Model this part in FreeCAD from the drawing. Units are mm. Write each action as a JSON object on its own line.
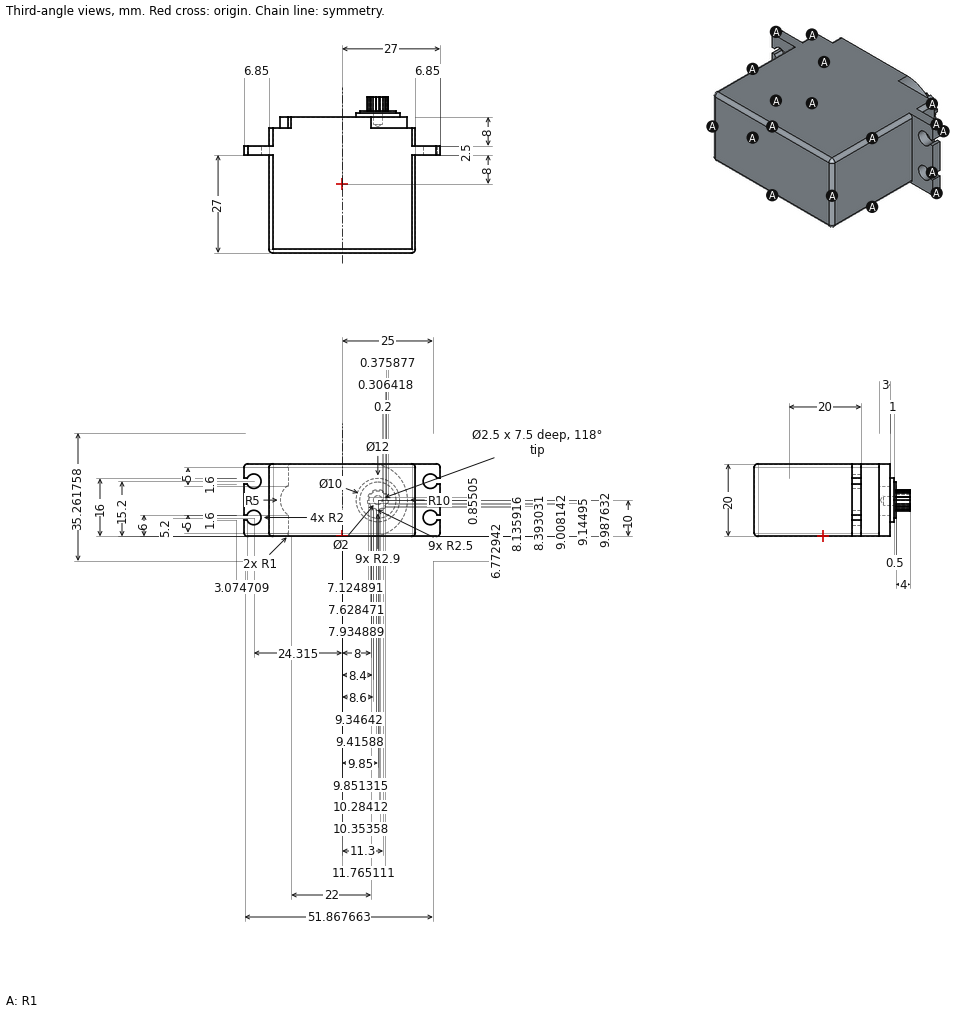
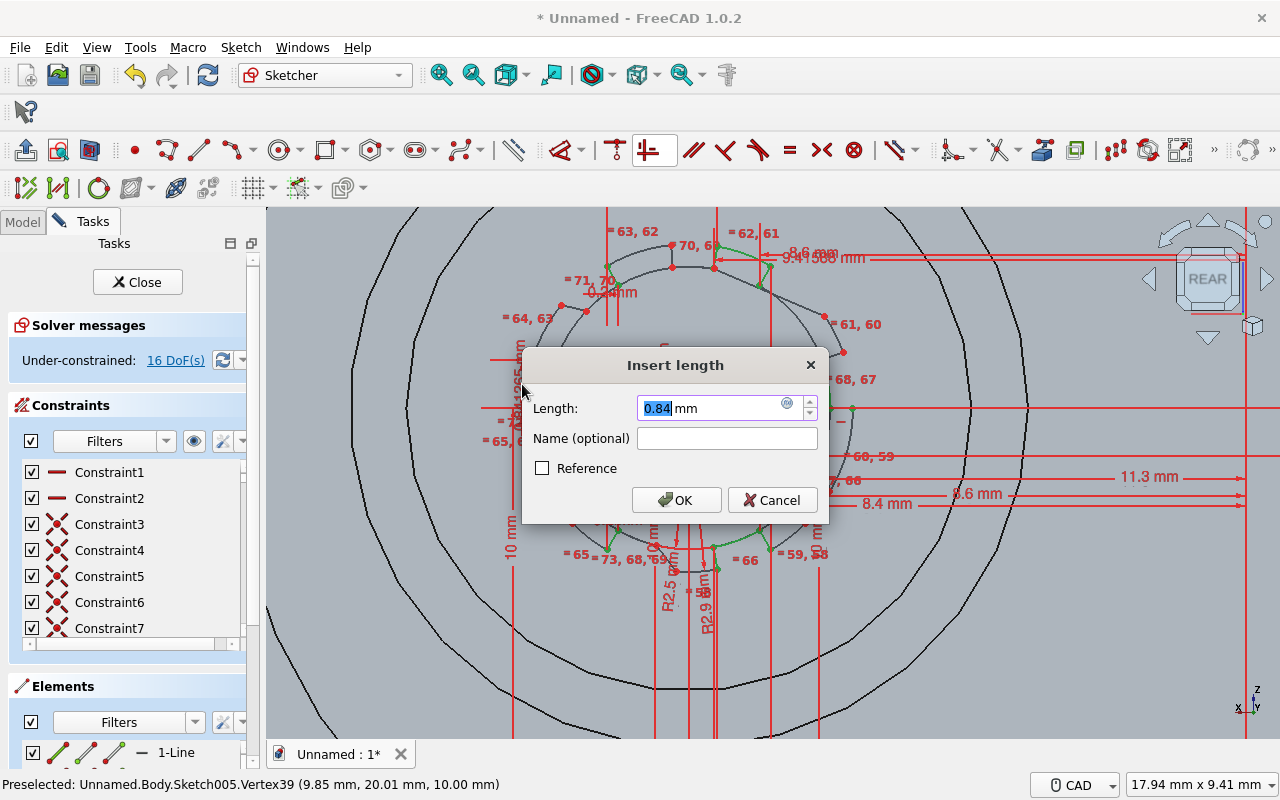
{"action": "type", "text": "0.85505"}
{"action": "key", "text": "Return"}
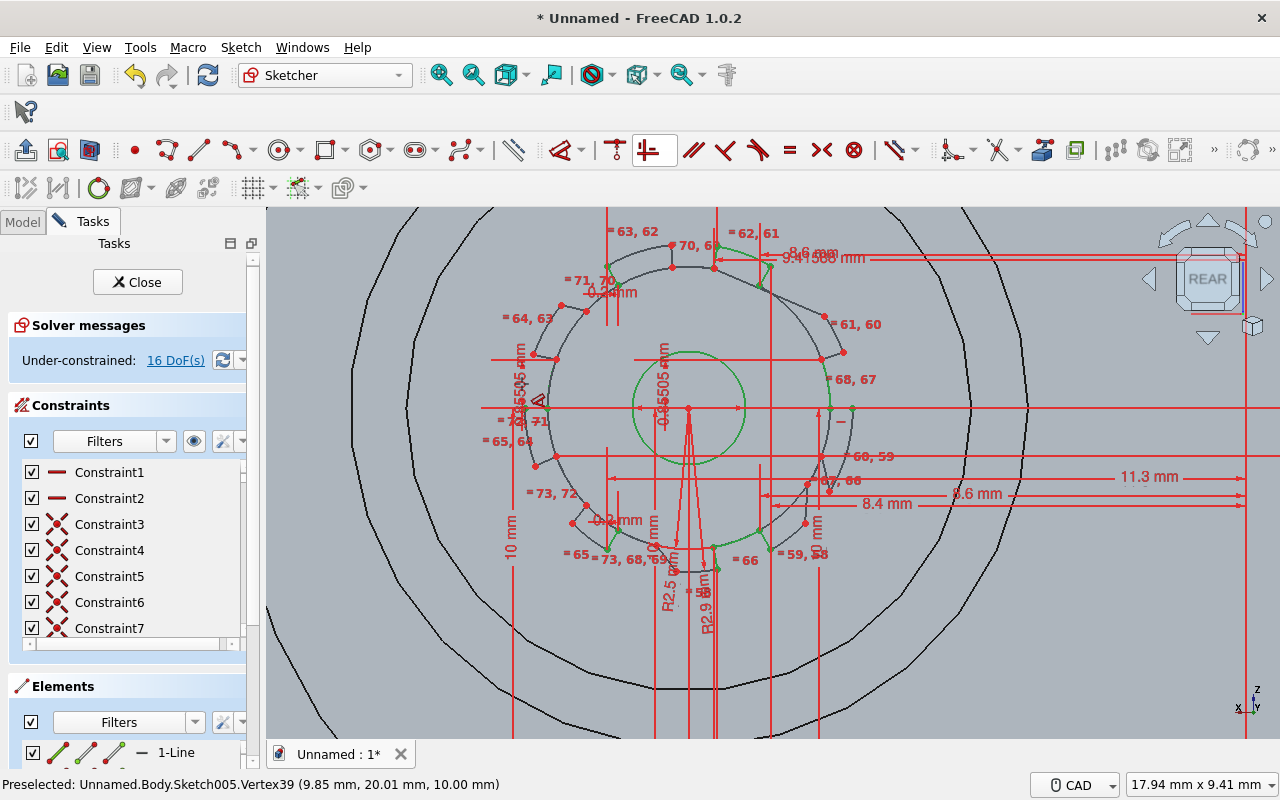
{"action": "left_click", "coordinate": [656, 546]}
{"action": "left_click", "coordinate": [725, 512]}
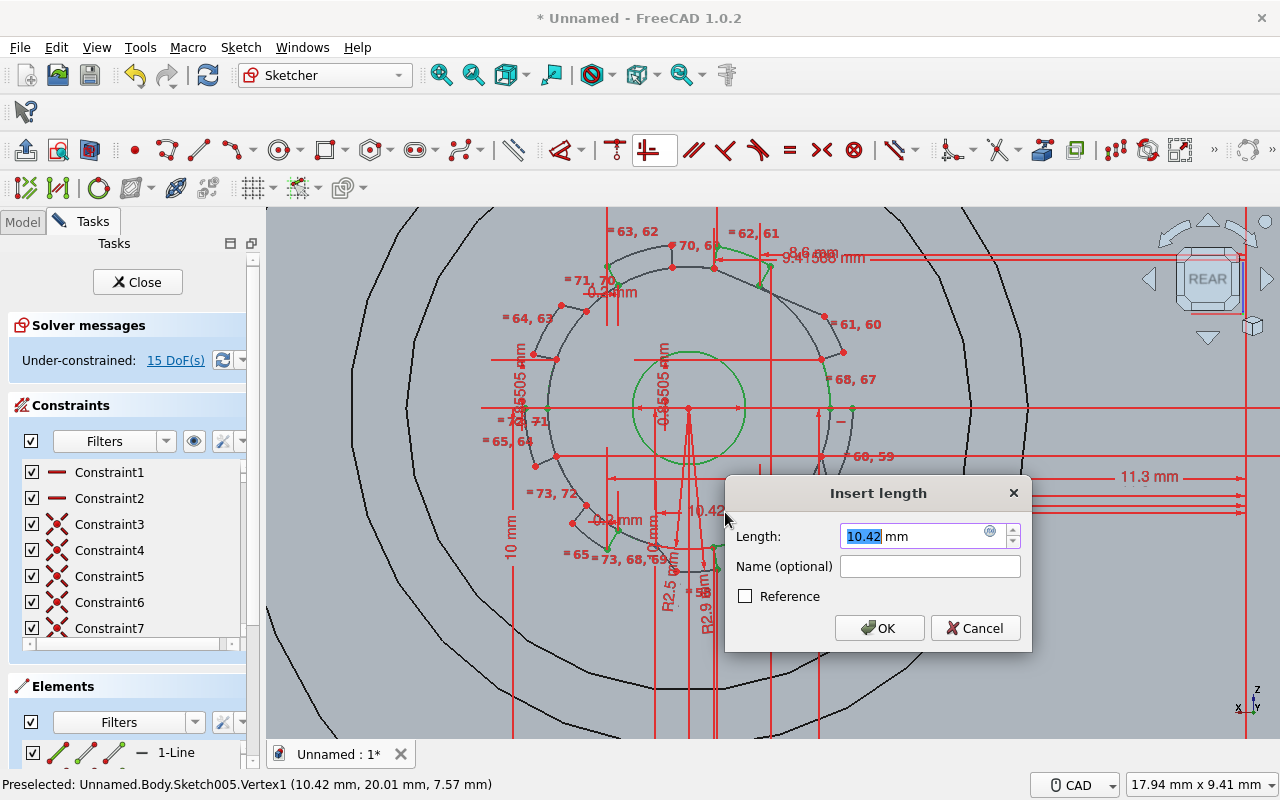
{"action": "type", "text": "10.28412"}
{"action": "key", "text": "Return"}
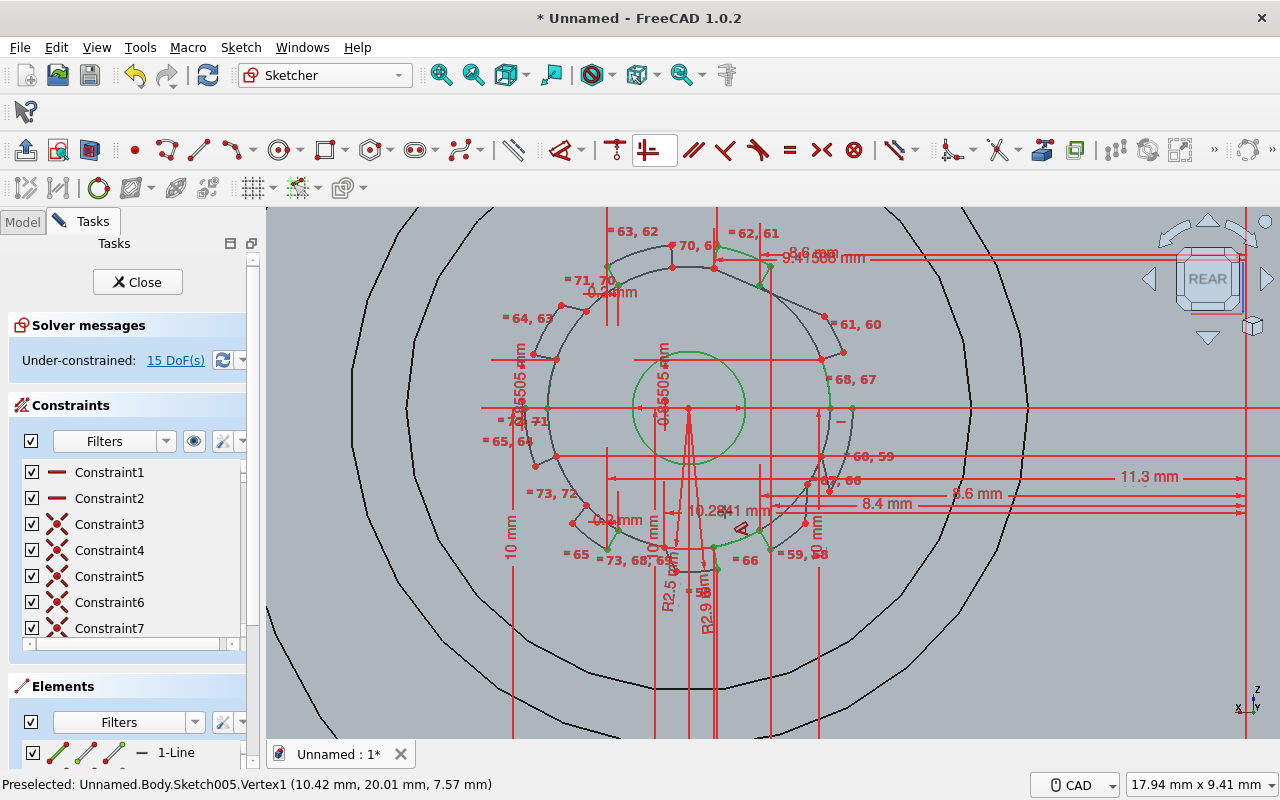
{"action": "left_click", "coordinate": [676, 571]}
{"action": "left_click", "coordinate": [896, 537]}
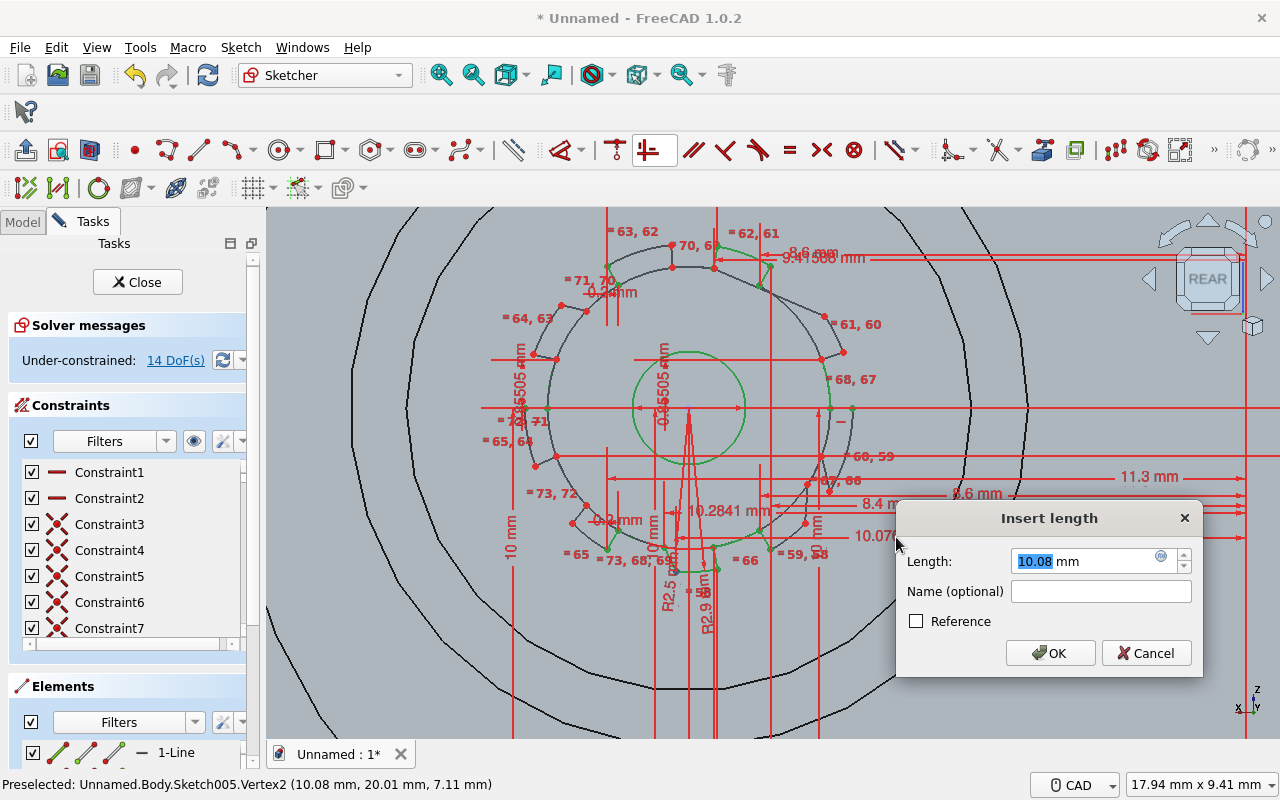
{"action": "type", "text": "10.35358"}
{"action": "key", "text": "Return"}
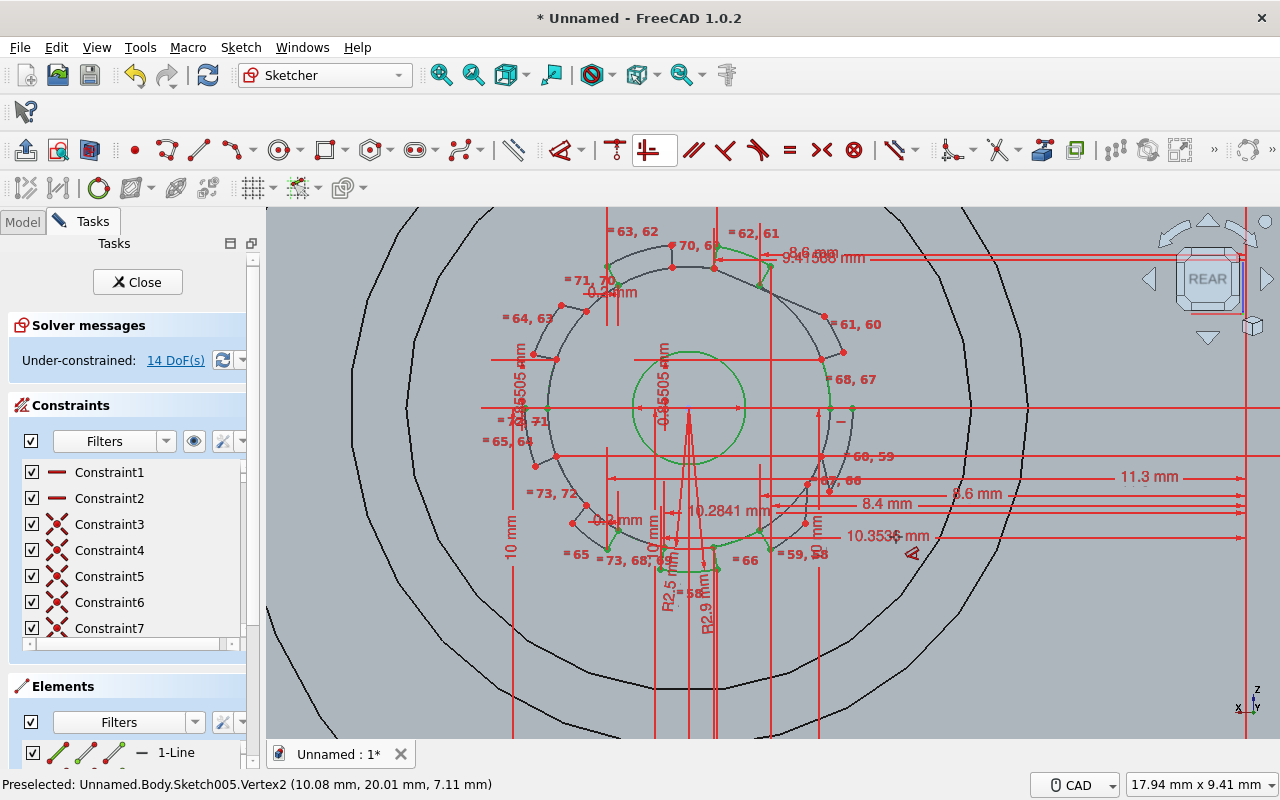
{"action": "left_click", "coordinate": [805, 524]}
{"action": "left_click", "coordinate": [1069, 490]}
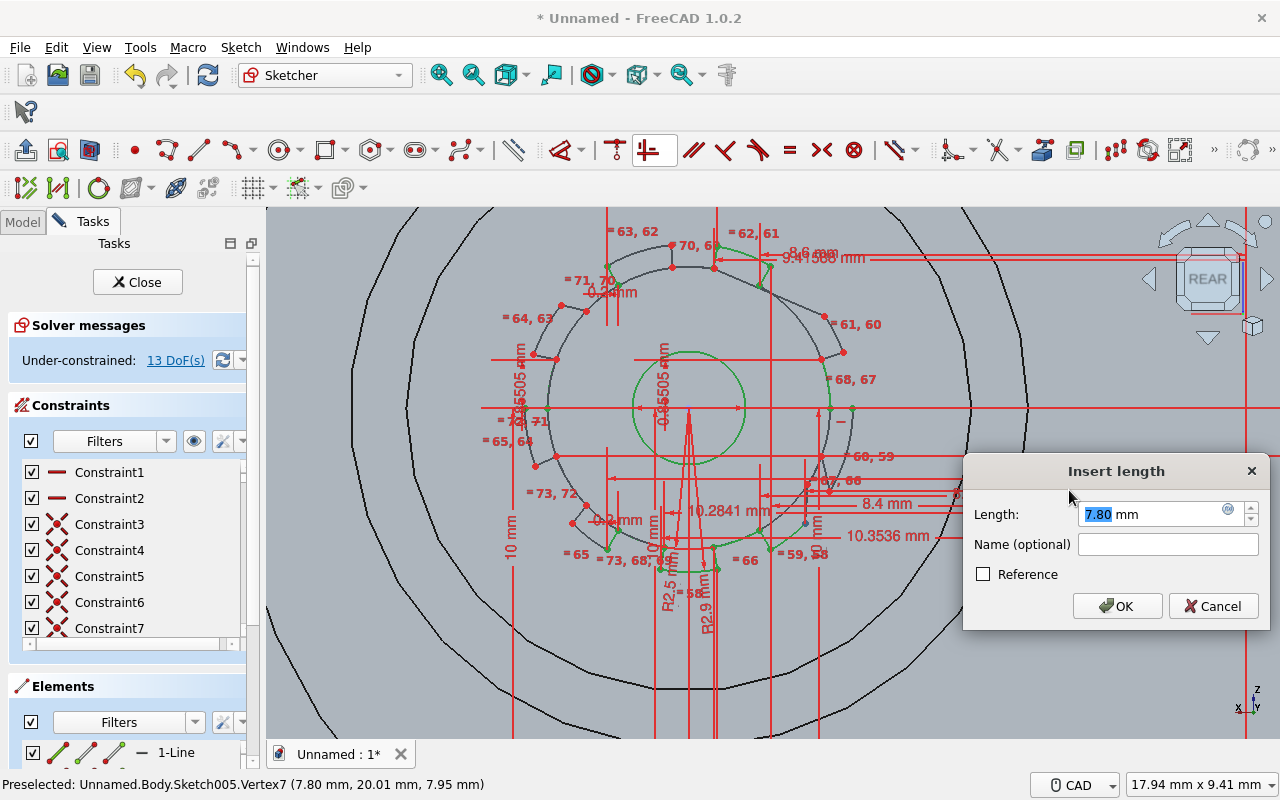
{"action": "type", "text": "7.628471"}
{"action": "key", "text": "Return"}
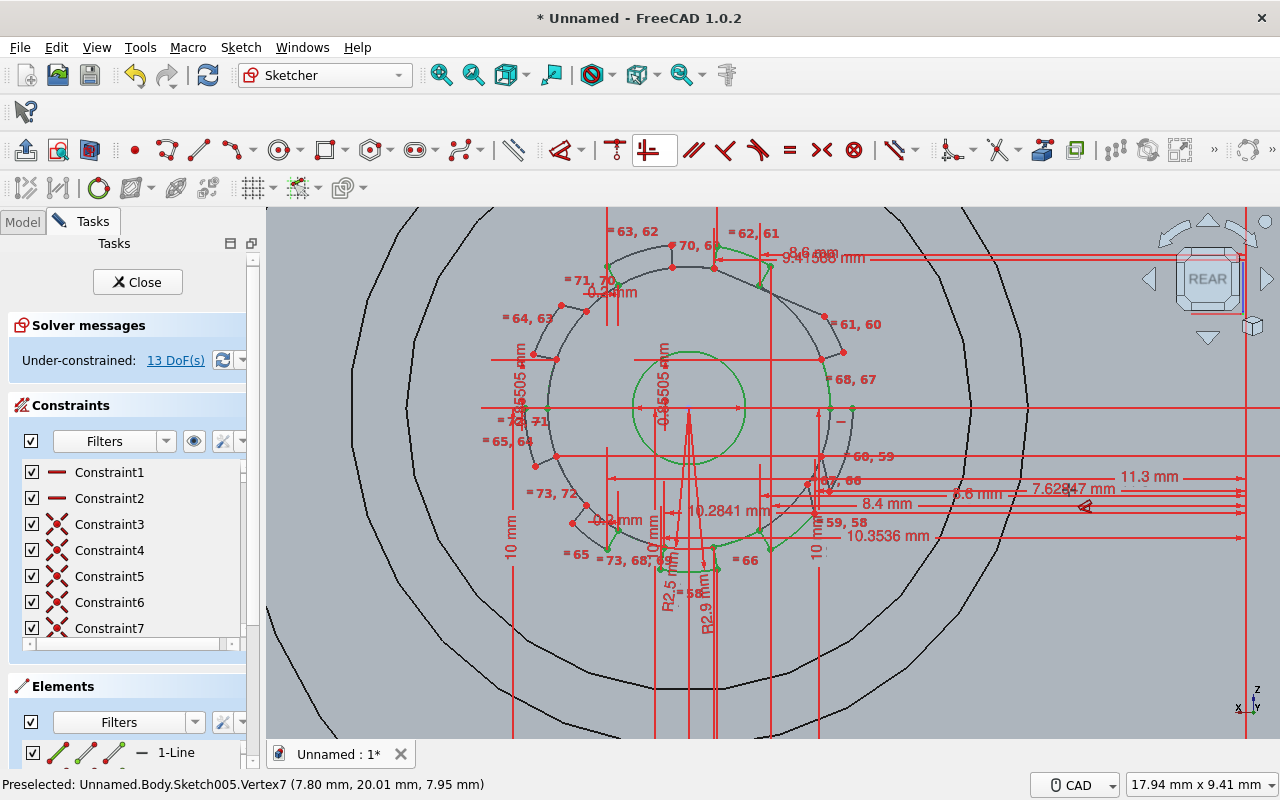
{"action": "left_click", "coordinate": [808, 485]}
{"action": "left_click", "coordinate": [961, 451]}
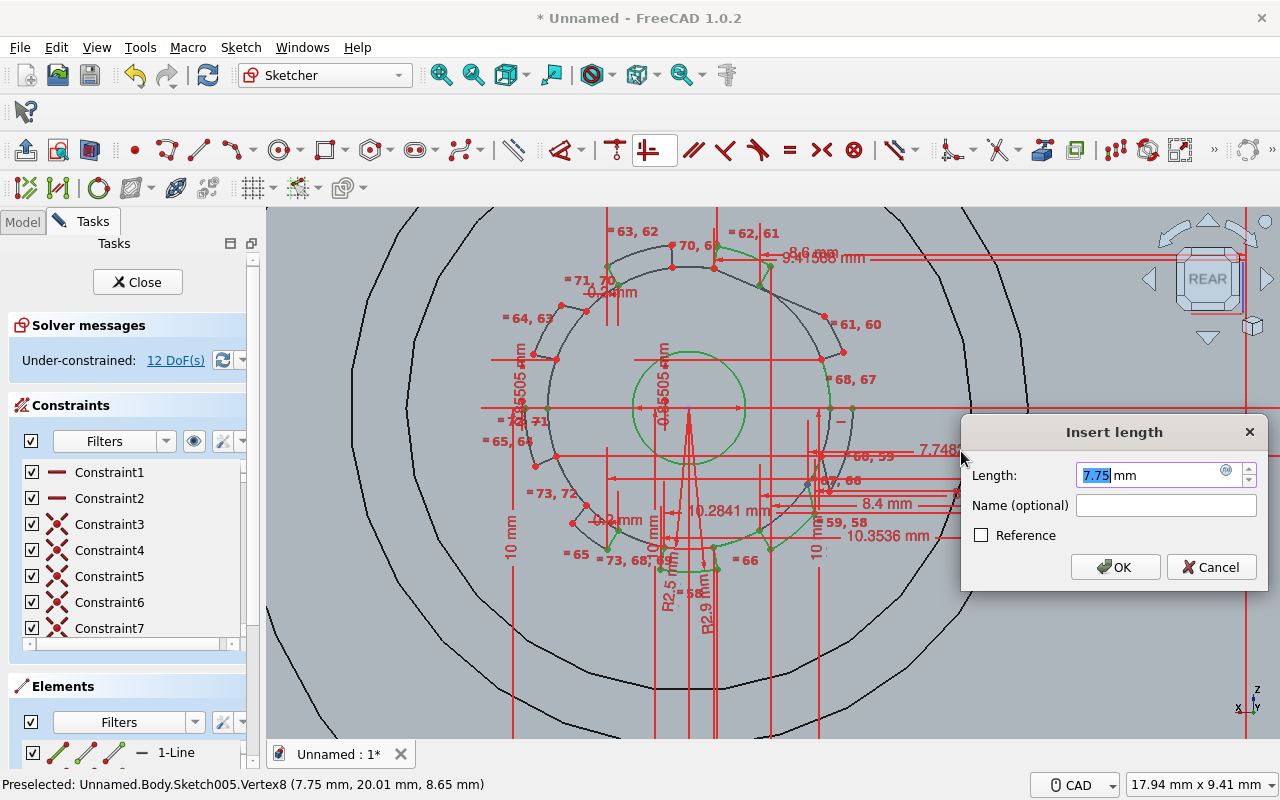
{"action": "type", "text": "7.934889"}
{"action": "key", "text": "Return"}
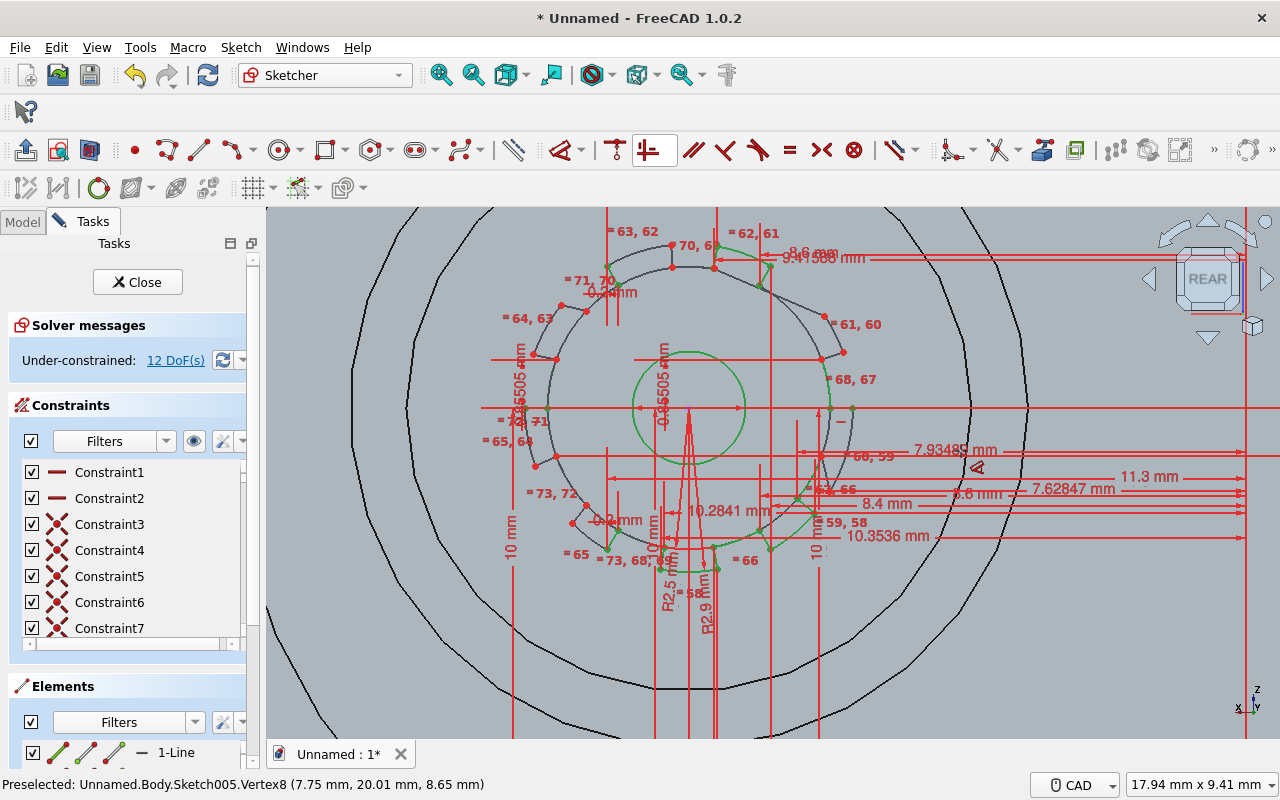
{"action": "left_click", "coordinate": [830, 492]}
{"action": "left_click", "coordinate": [1038, 458]}